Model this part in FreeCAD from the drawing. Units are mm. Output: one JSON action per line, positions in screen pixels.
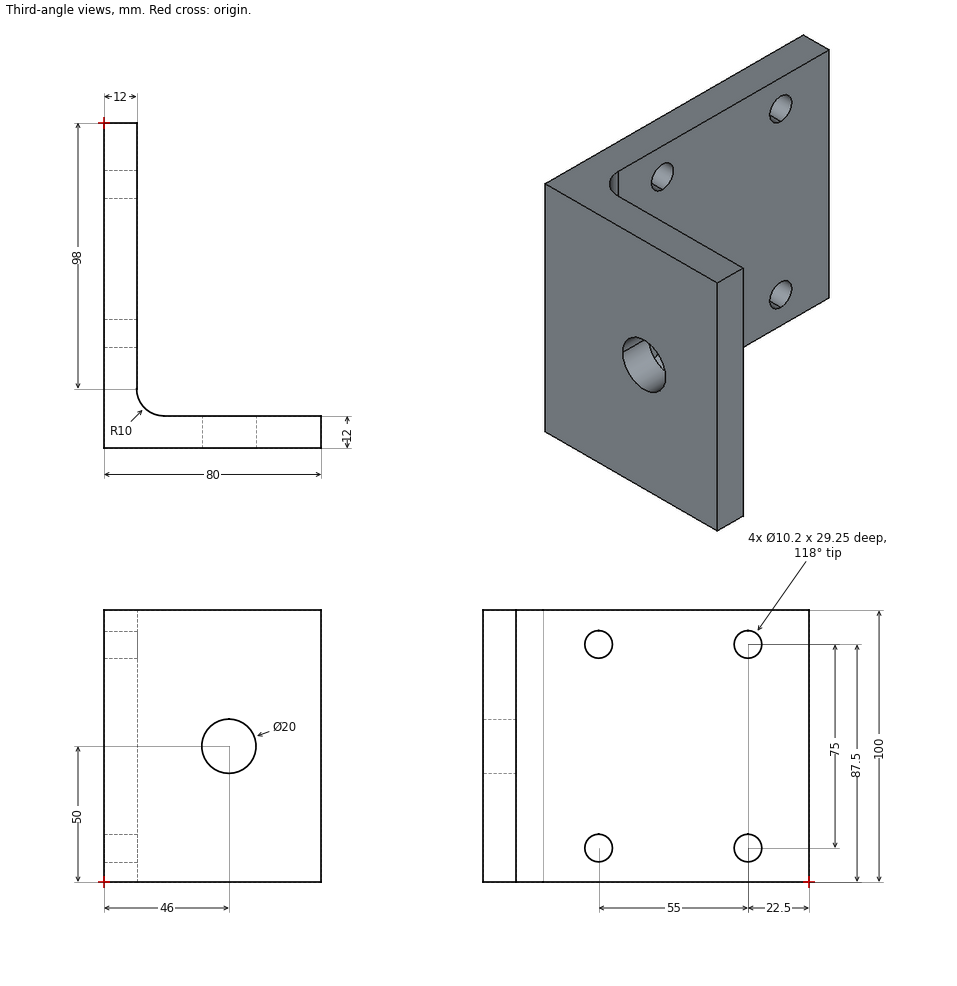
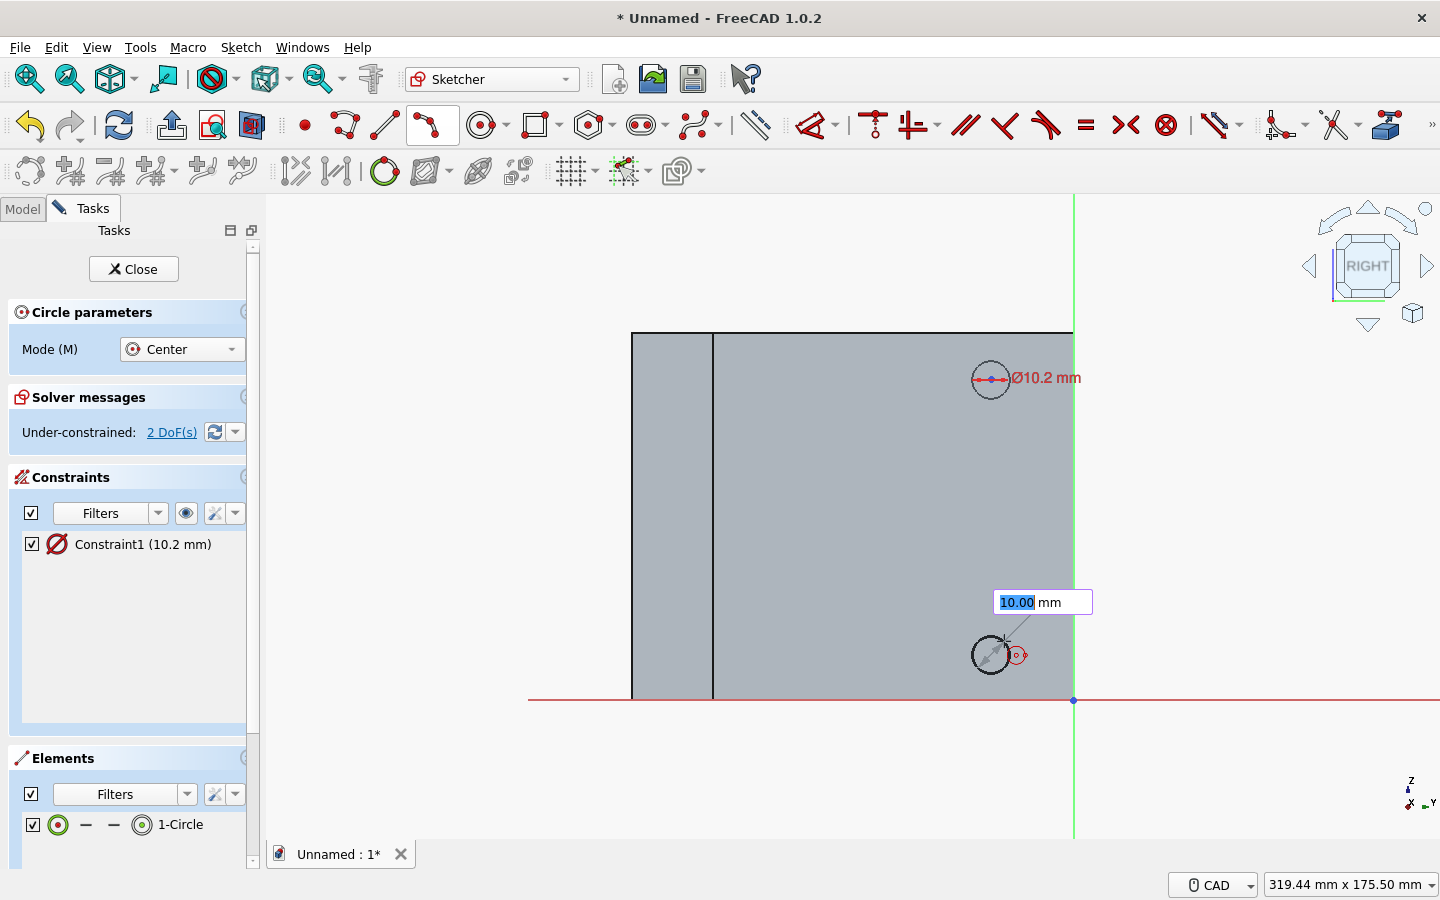
{"action": "type", "text": "10.2"}
{"action": "key", "text": "Return"}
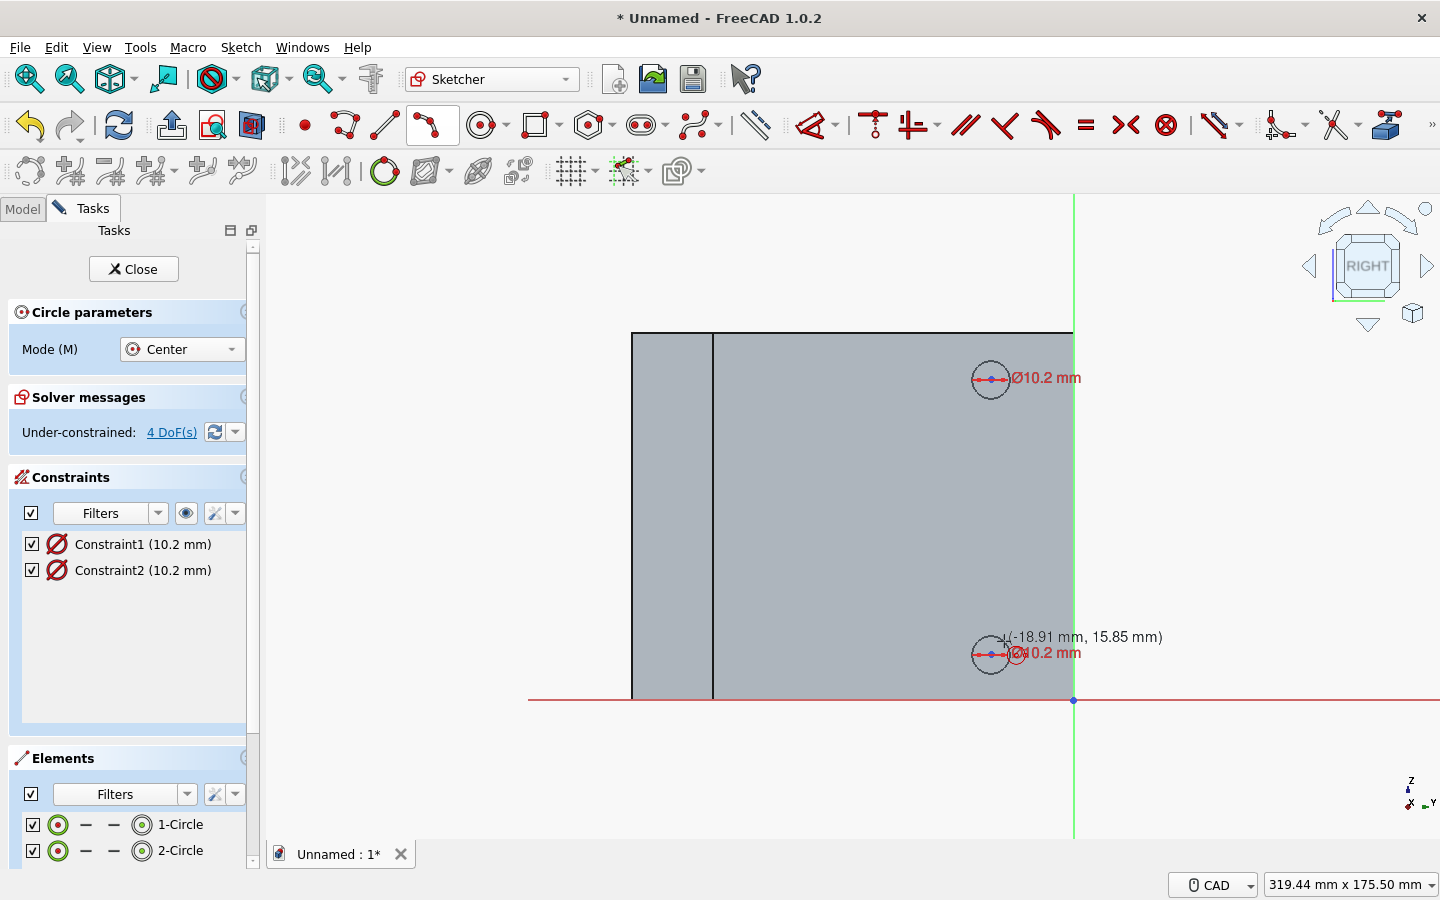
{"action": "left_click", "coordinate": [789, 654]}
{"action": "mouse_move", "coordinate": [802, 641]}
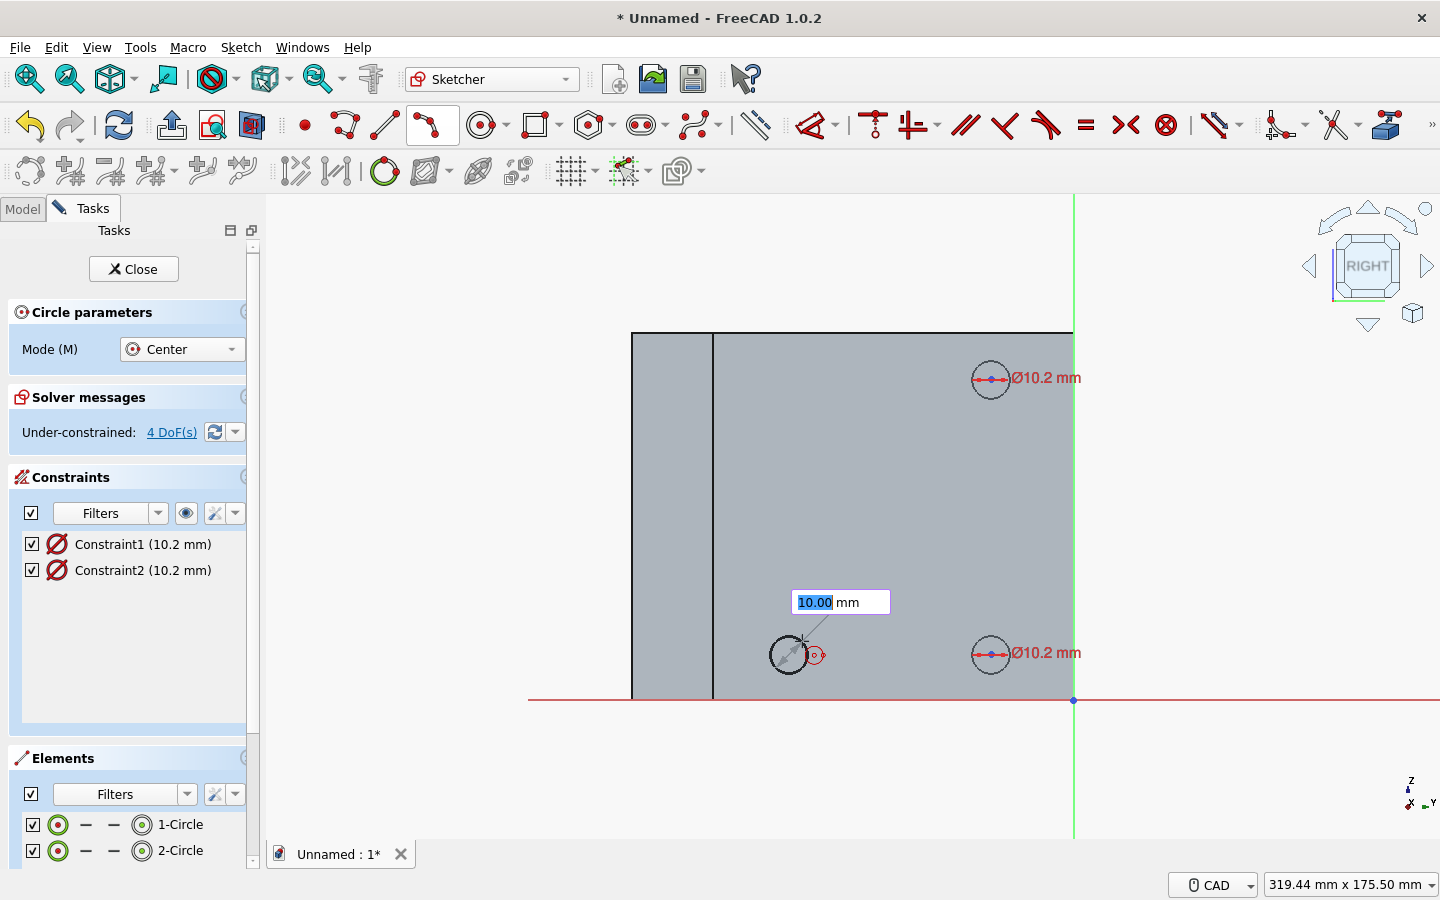
{"action": "type", "text": "10.2"}
{"action": "key", "text": "Return"}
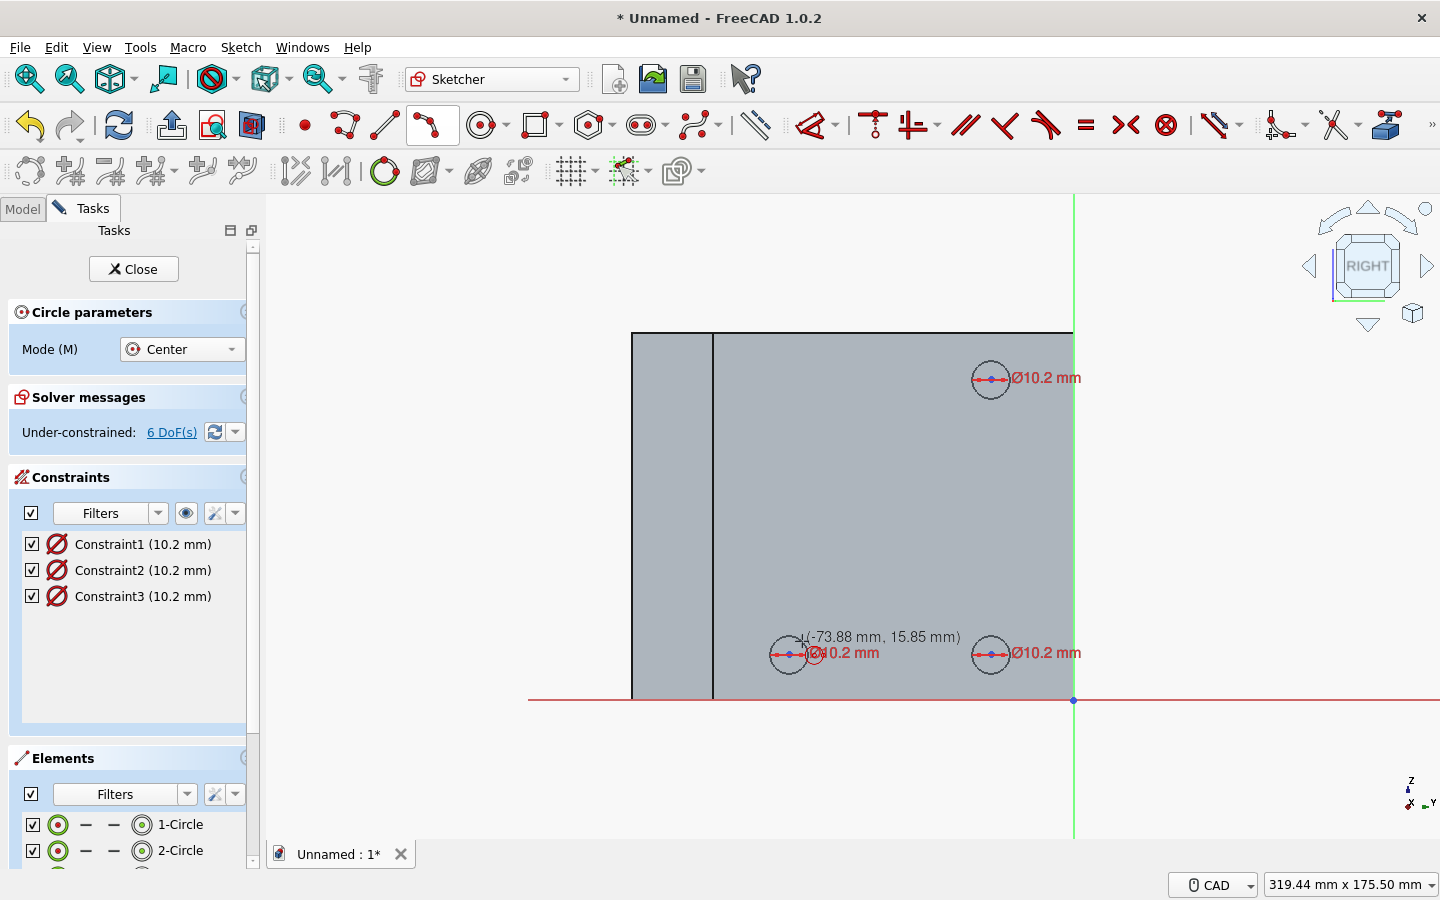
{"action": "left_click", "coordinate": [789, 379]}
{"action": "mouse_move", "coordinate": [802, 365]}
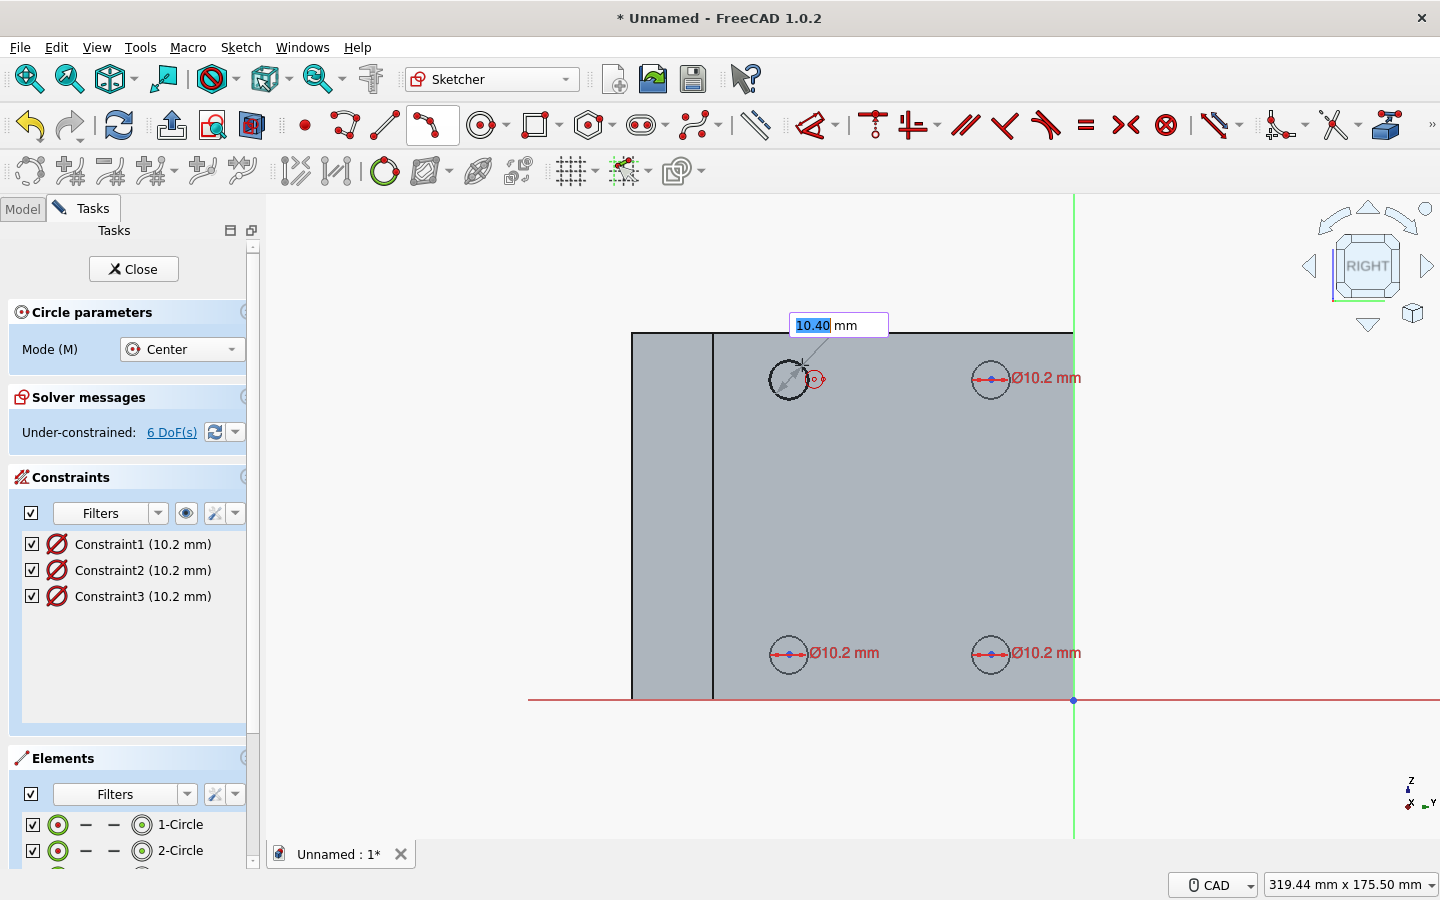
{"action": "type", "text": "10.2"}
{"action": "key", "text": "Return"}
{"action": "key", "text": "Escape"}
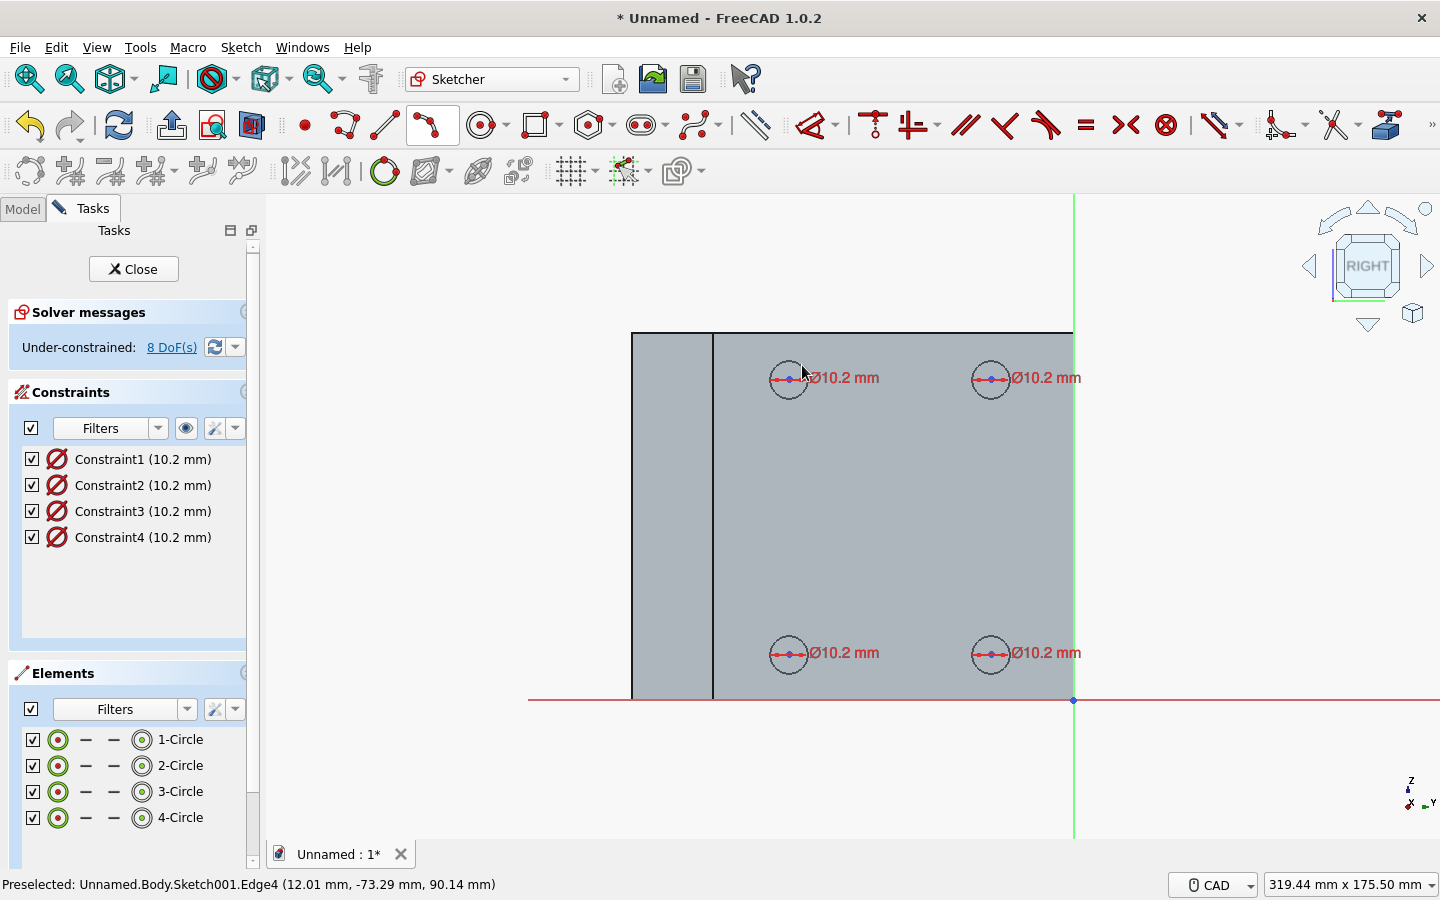
{"action": "left_click", "coordinate": [810, 126]}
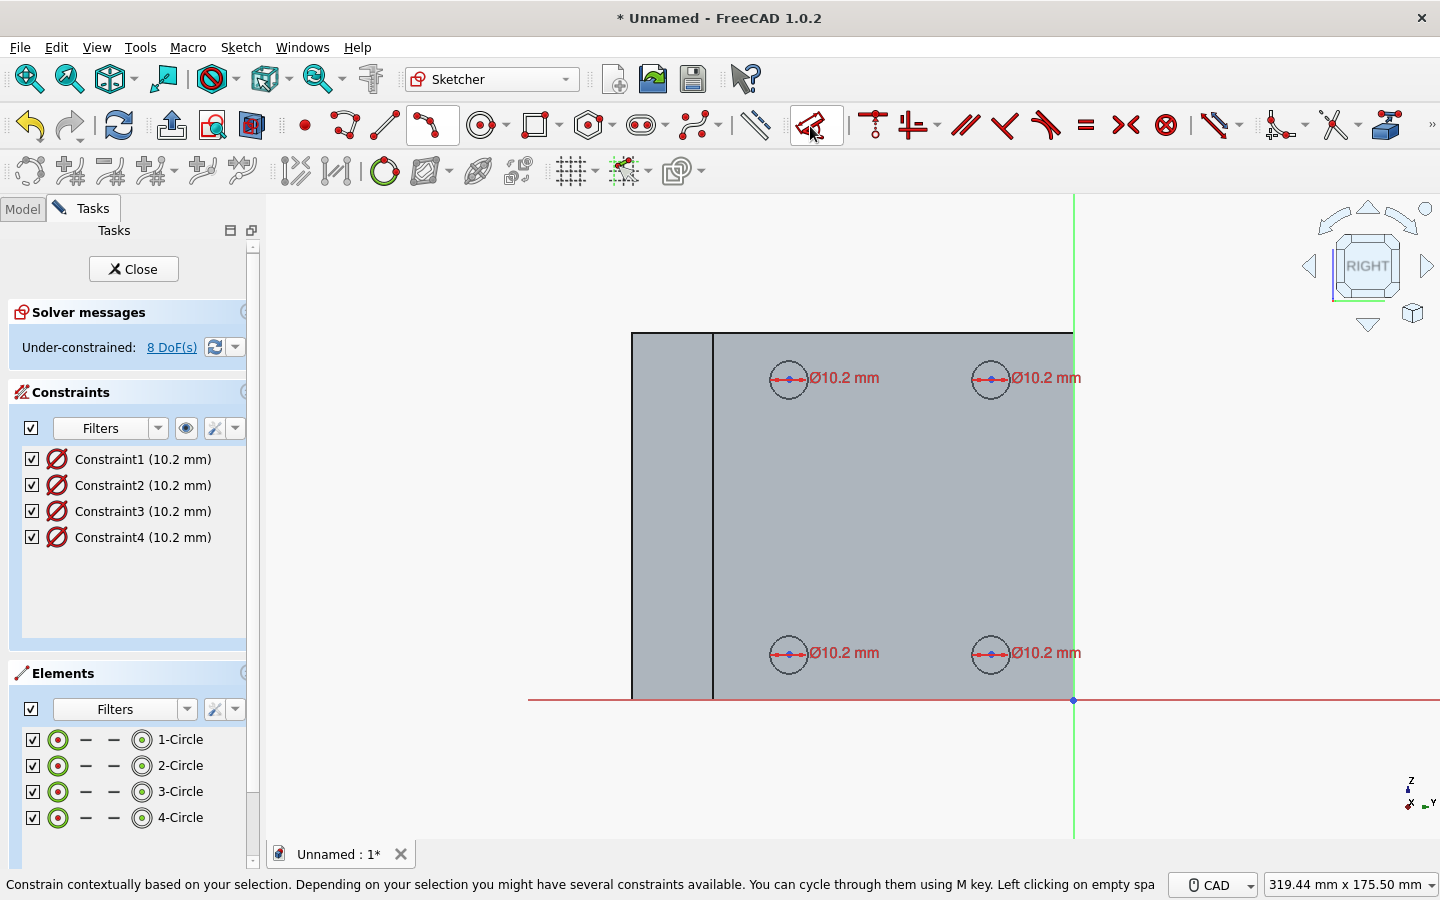
{"action": "left_click", "coordinate": [991, 380]}